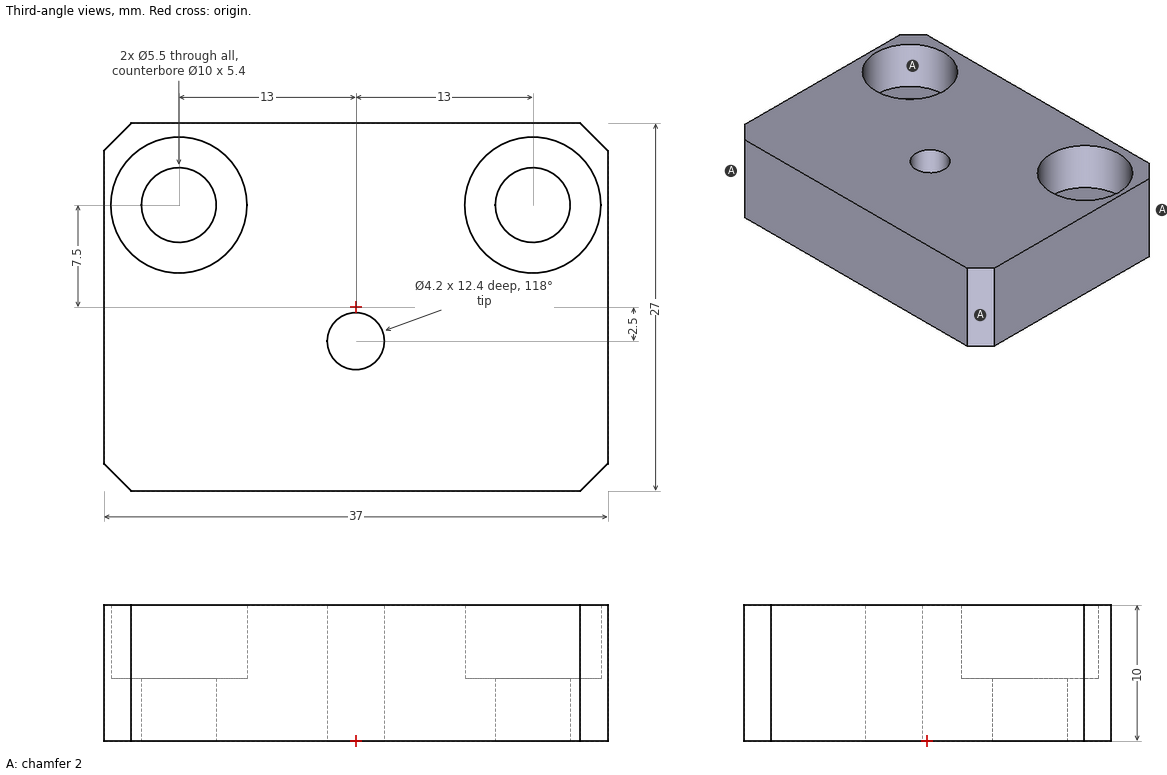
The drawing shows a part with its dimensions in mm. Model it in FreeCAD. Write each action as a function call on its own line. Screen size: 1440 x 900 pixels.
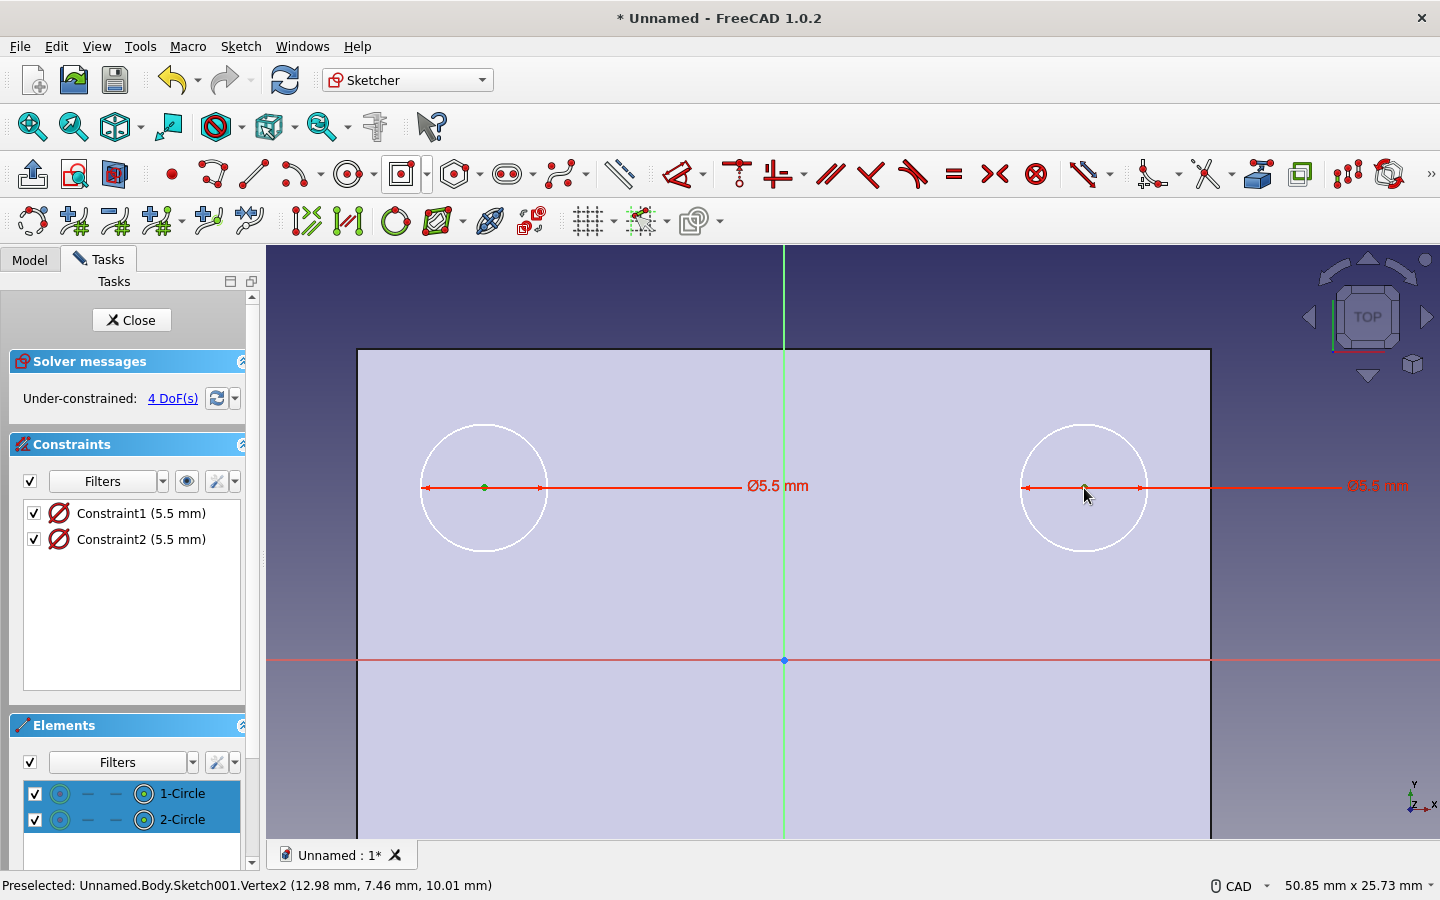
key(h)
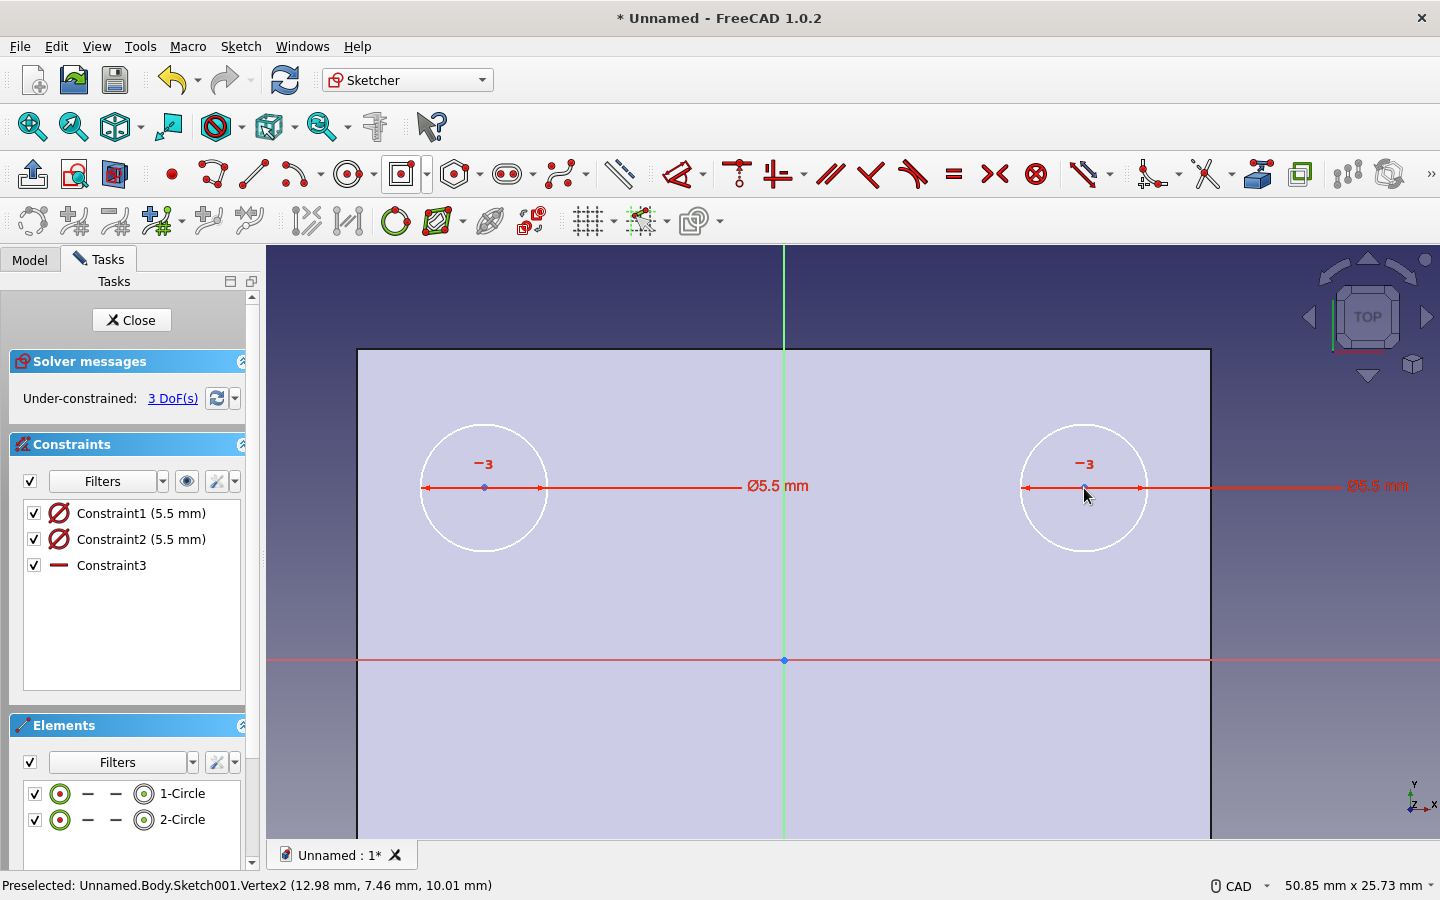
click(676, 174)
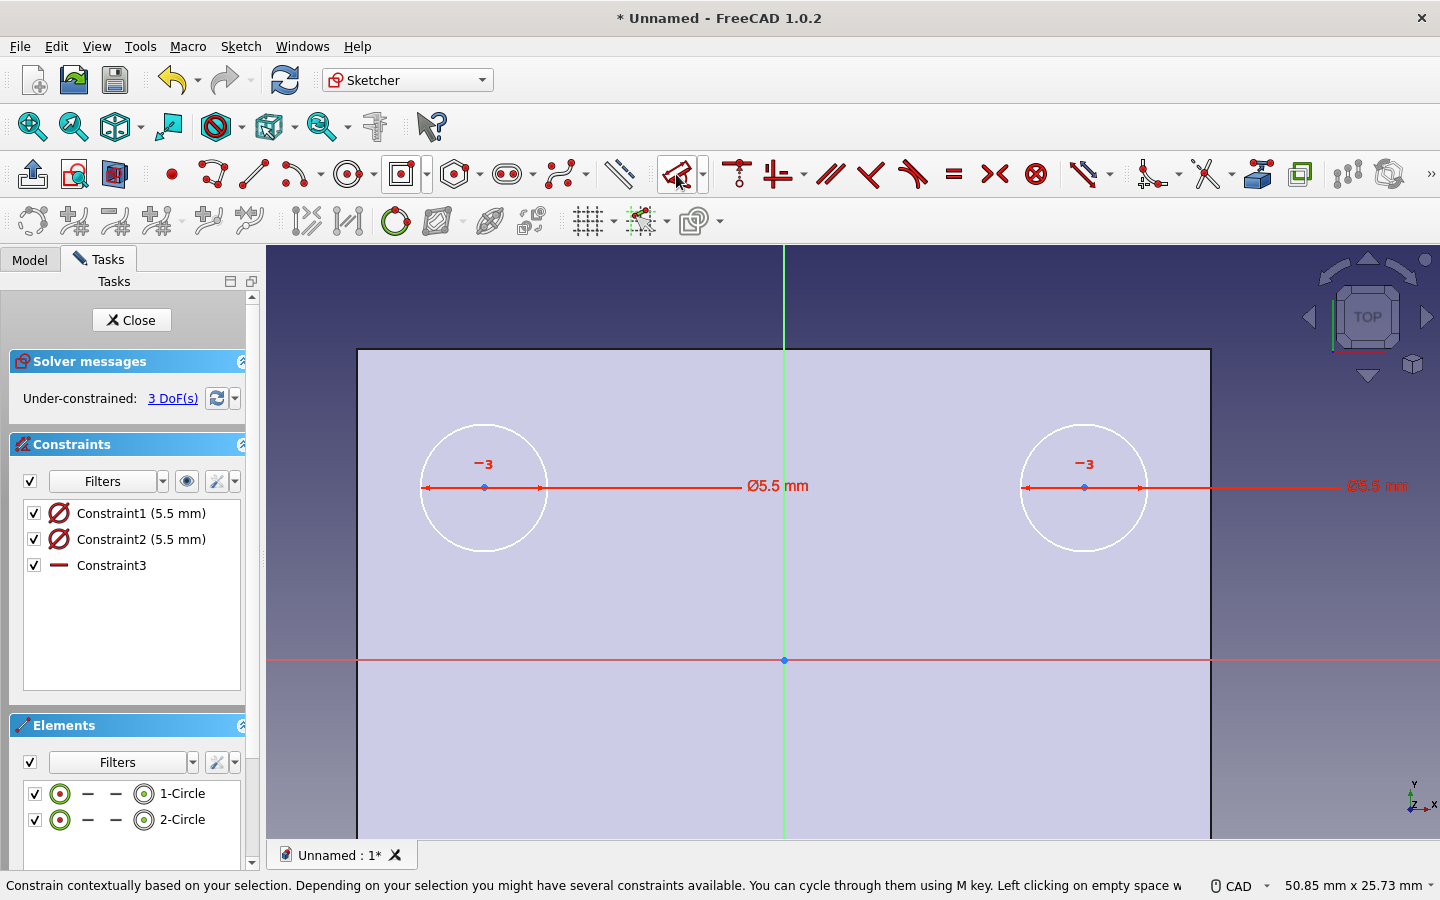
click(484, 488)
click(634, 694)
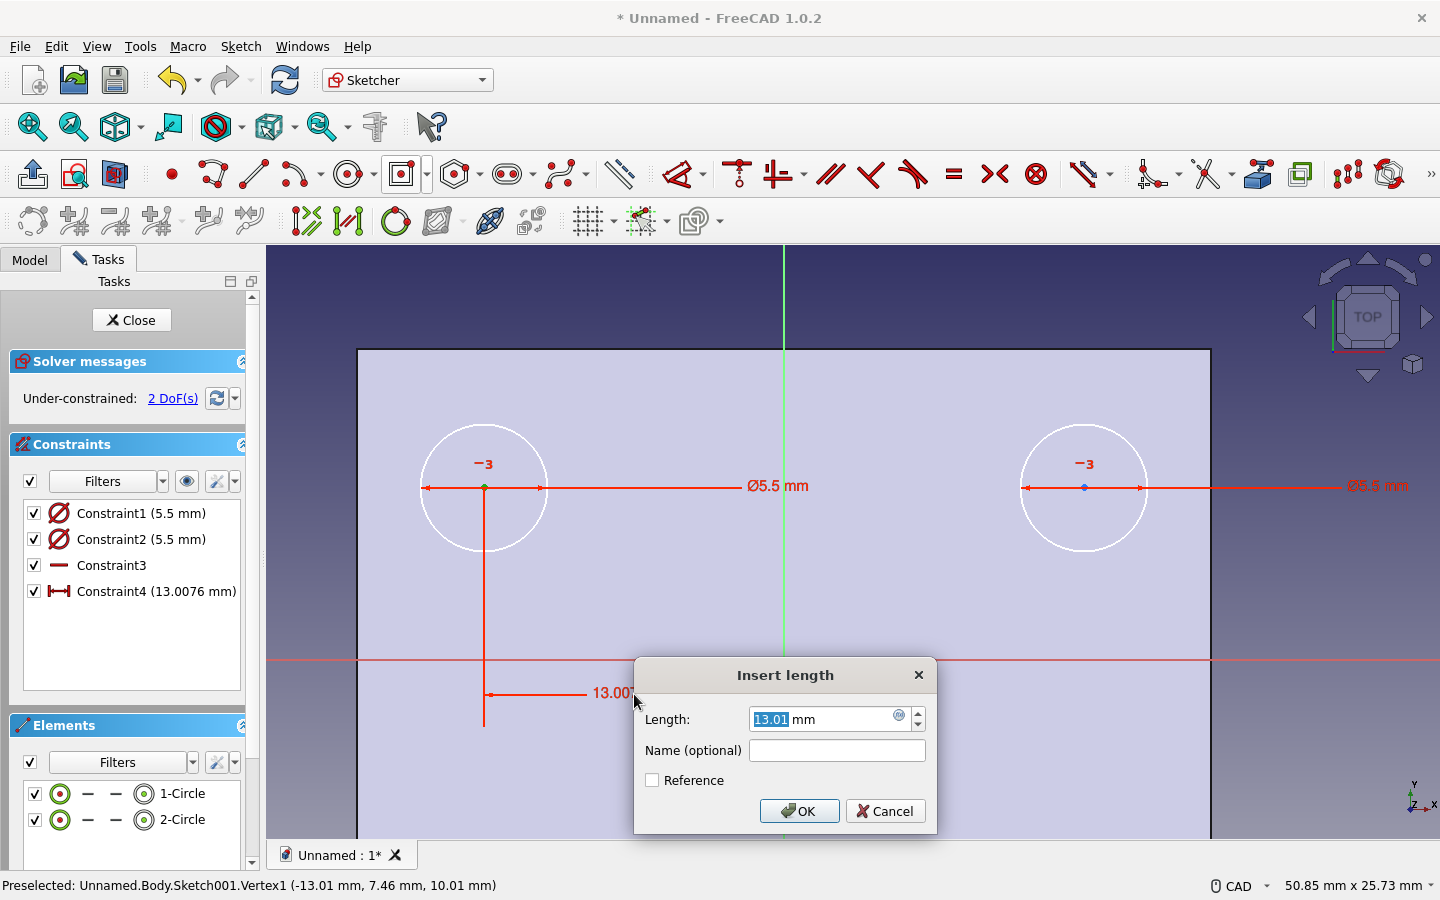
text(13)
key(Return)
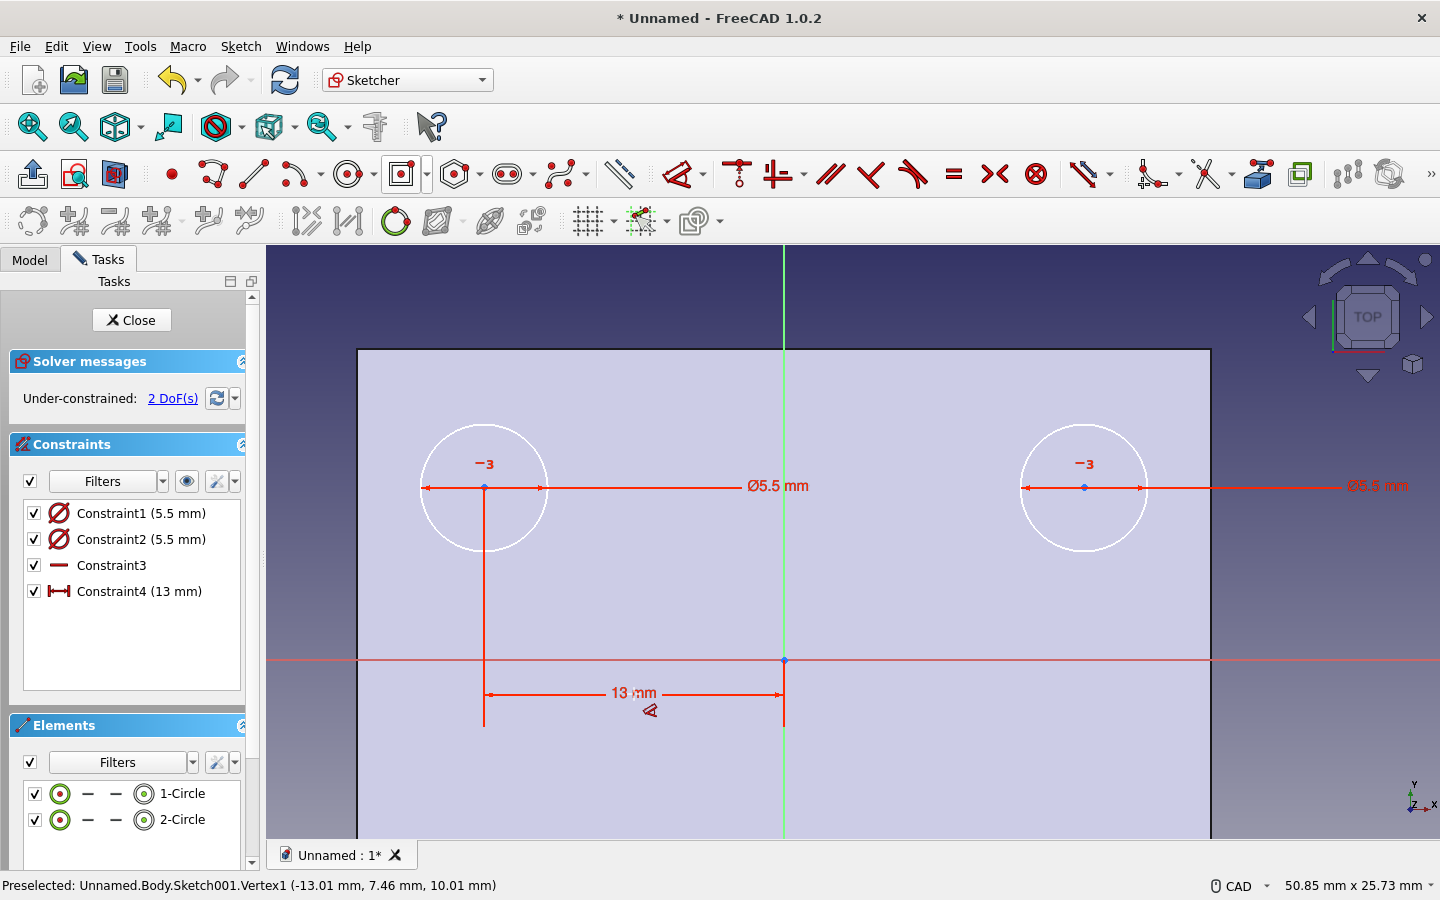
click(1084, 488)
click(934, 694)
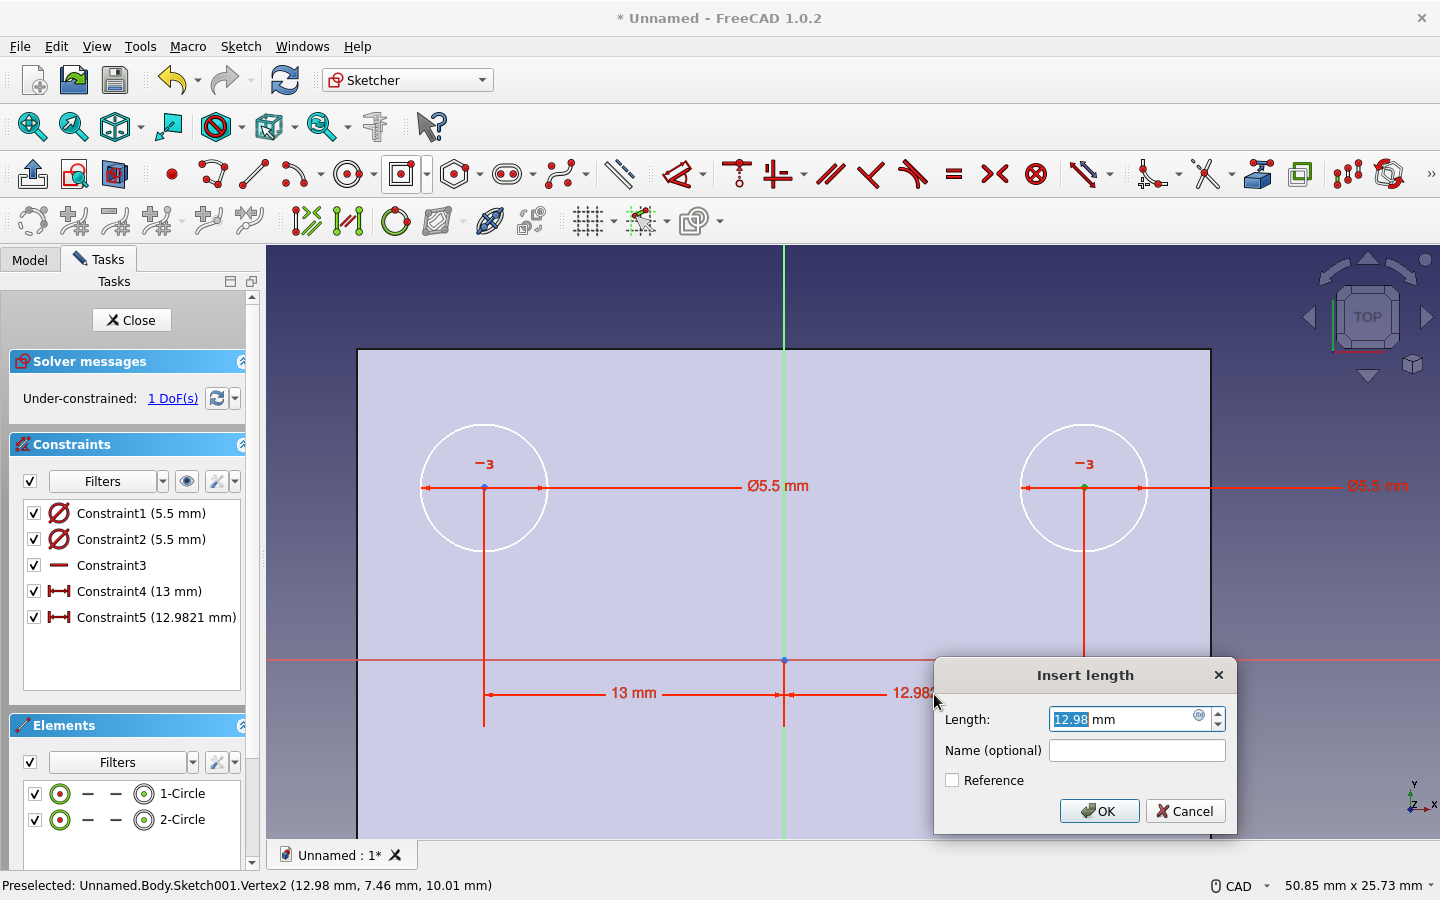
text(13)
key(Return)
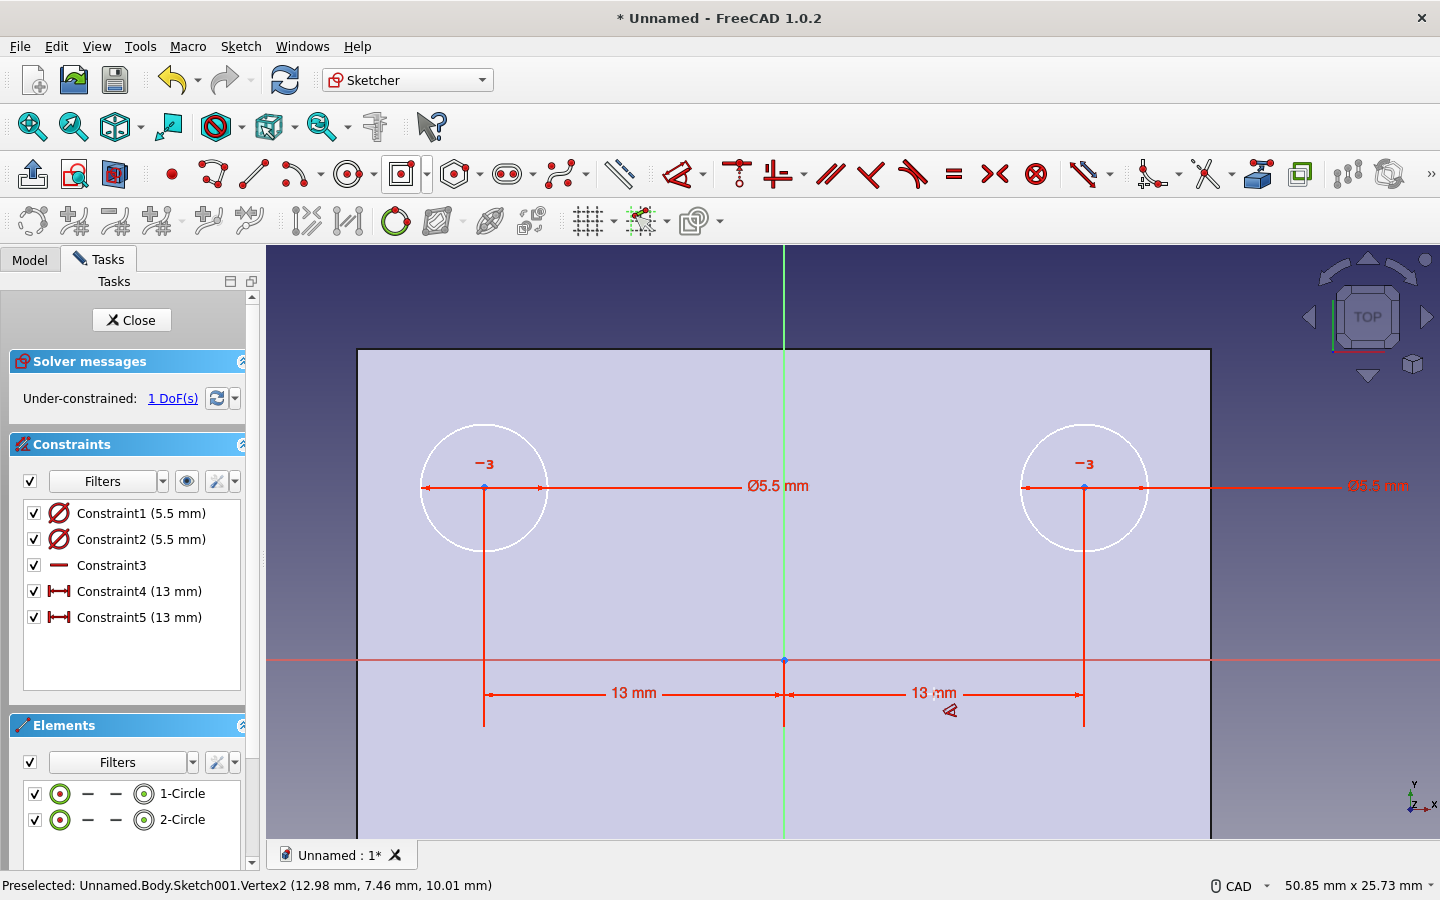
click(484, 488)
click(450, 574)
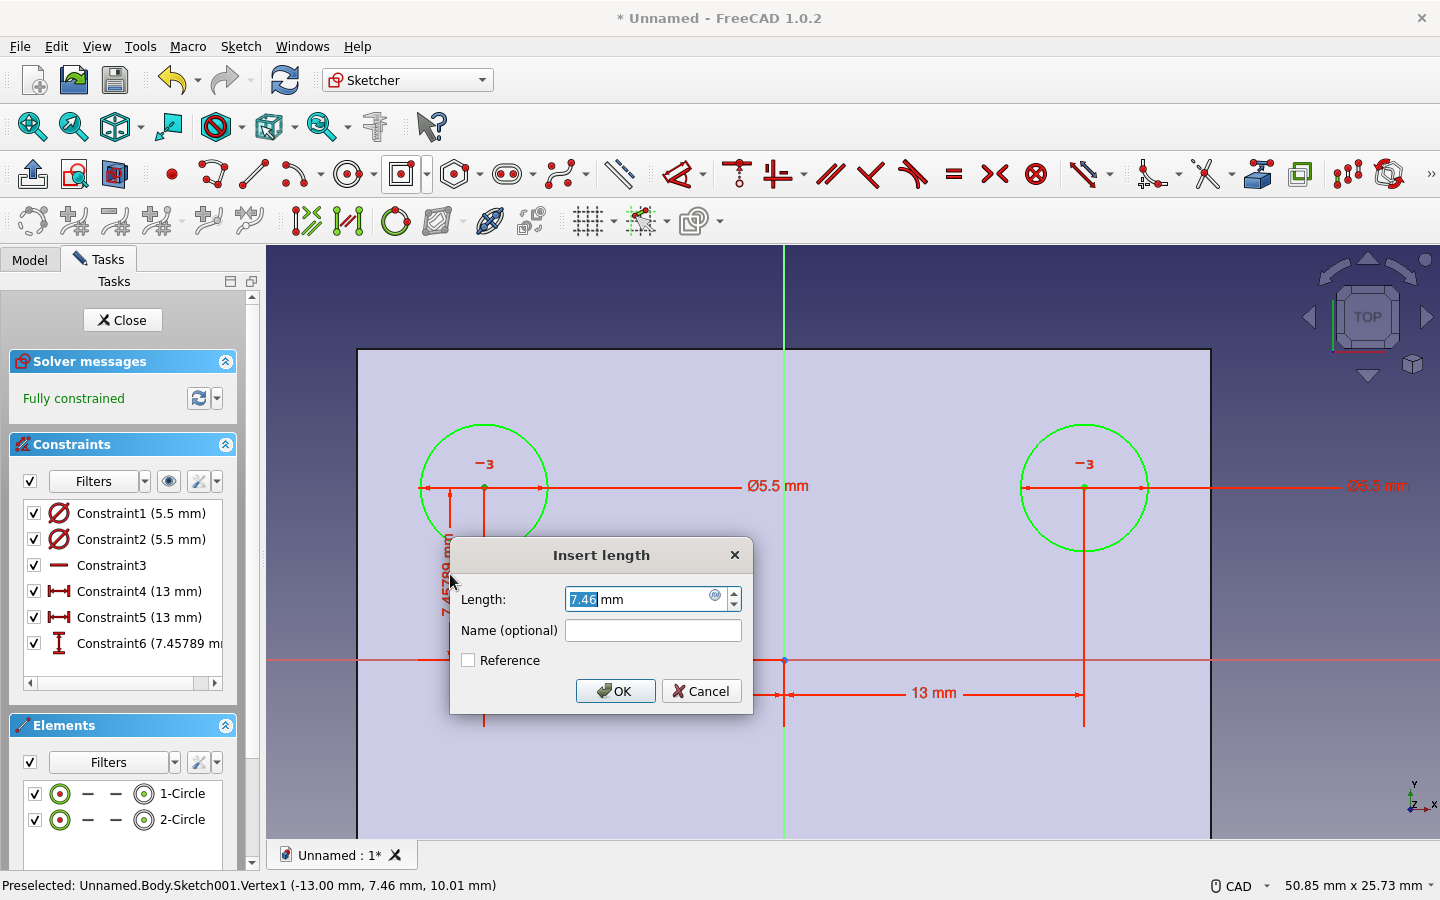
text(7.5)
key(Return)
key(Escape)